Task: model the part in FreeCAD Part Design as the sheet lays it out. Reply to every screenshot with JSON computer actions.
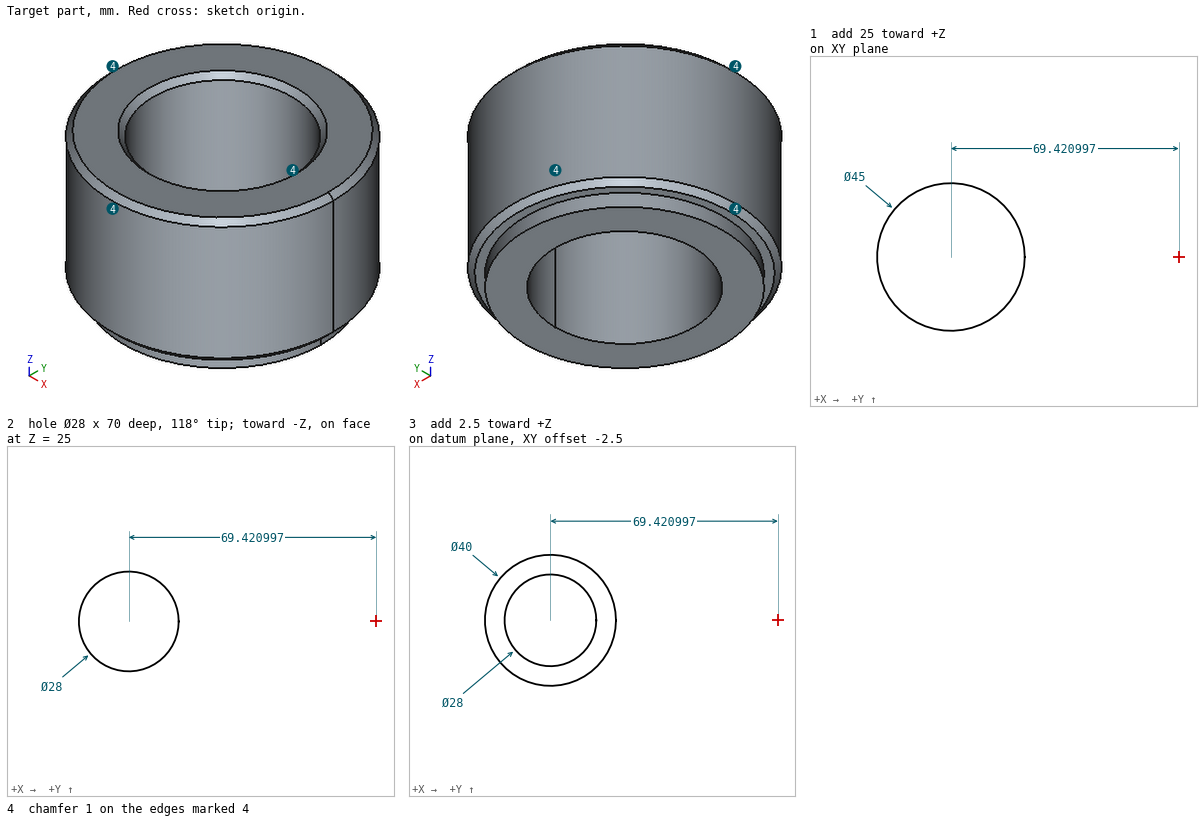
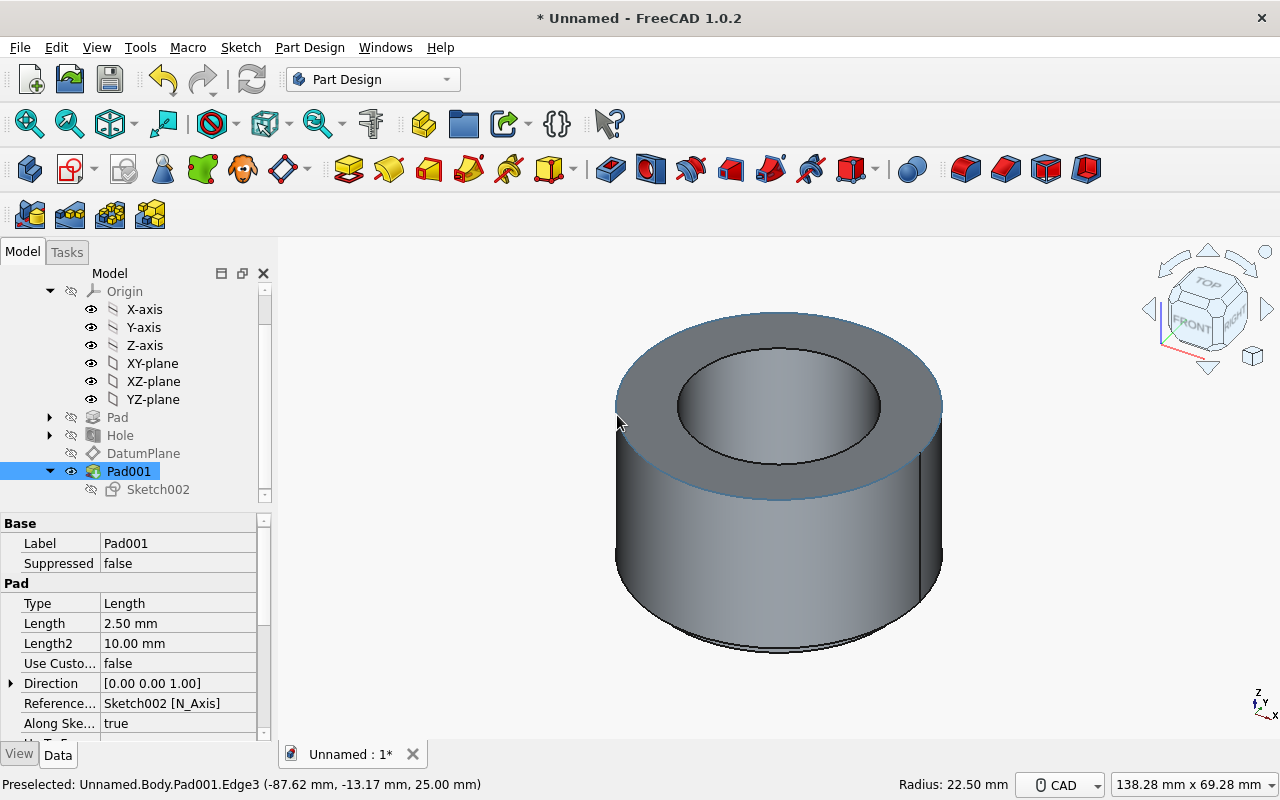
{"action": "left_click", "coordinate": [691, 376], "text": "ctrl"}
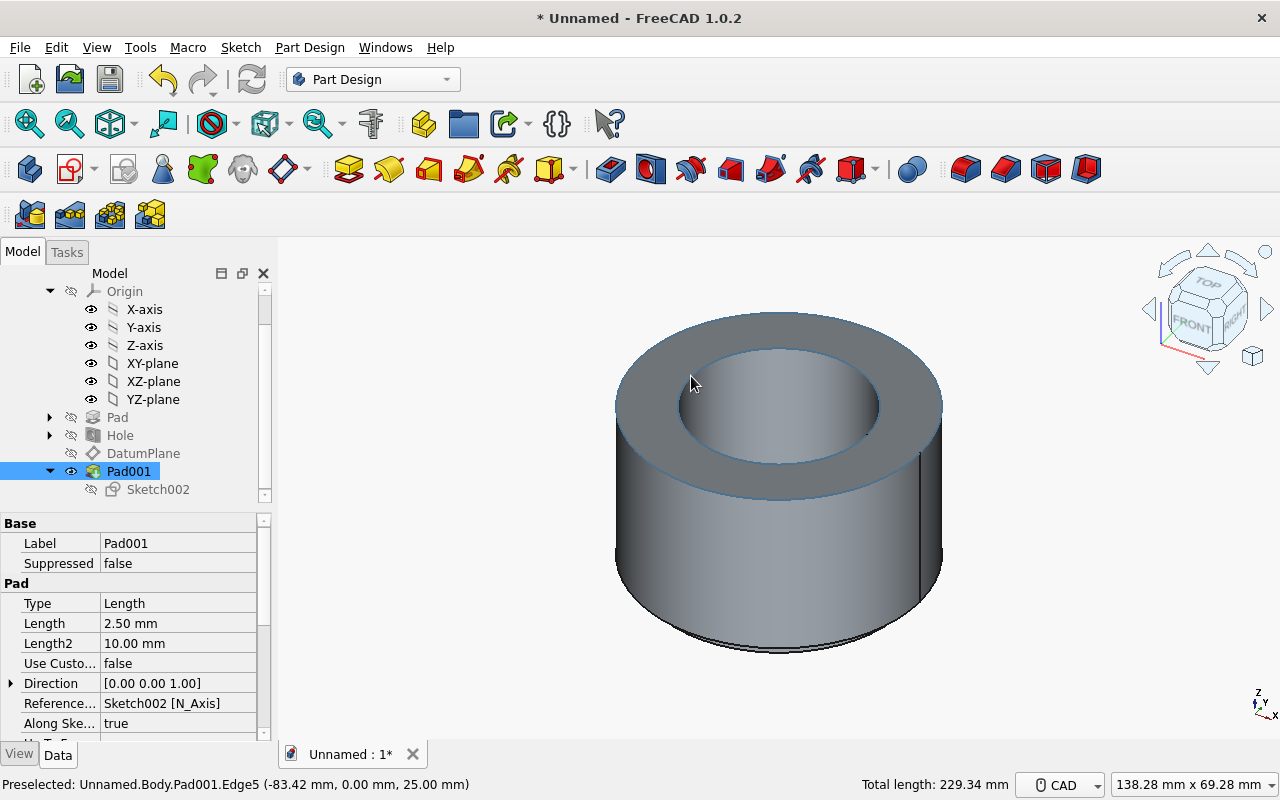
{"action": "key", "text": "0"}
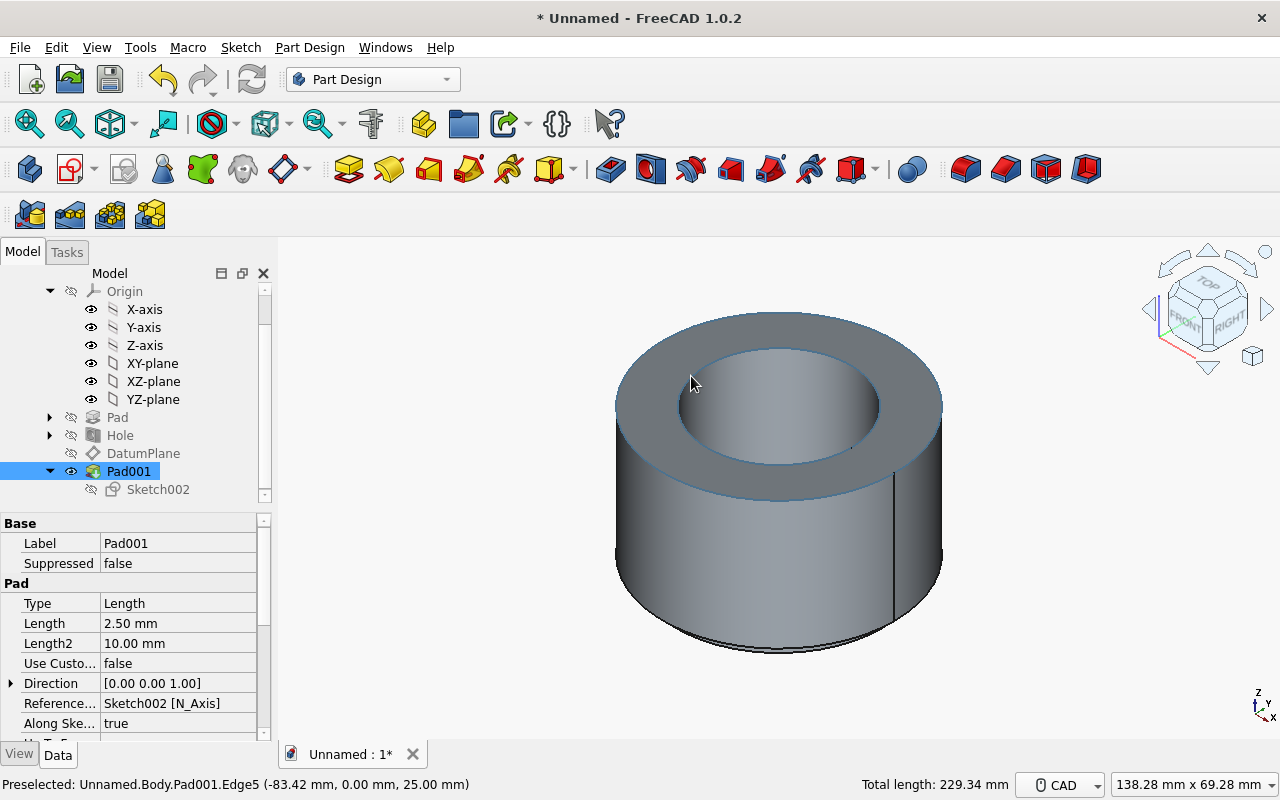
{"action": "key", "text": "2"}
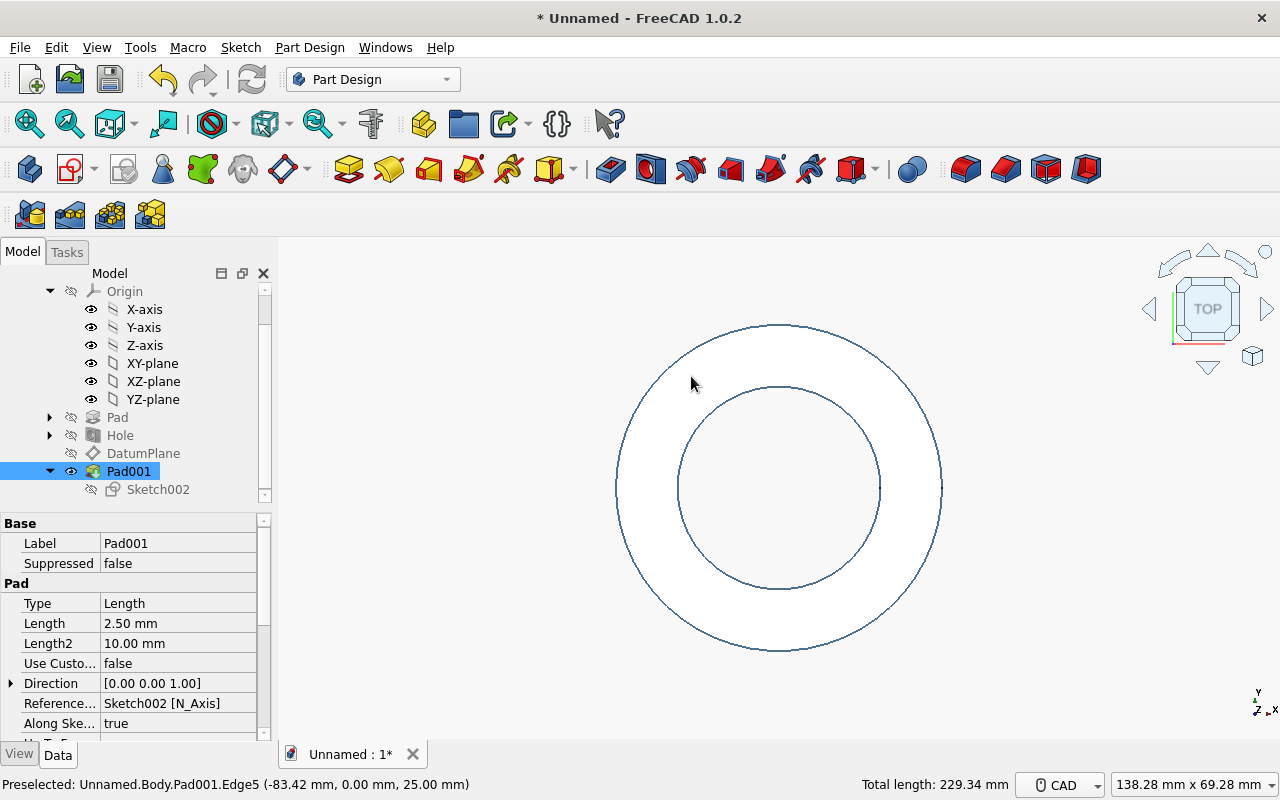
{"action": "key", "text": "1"}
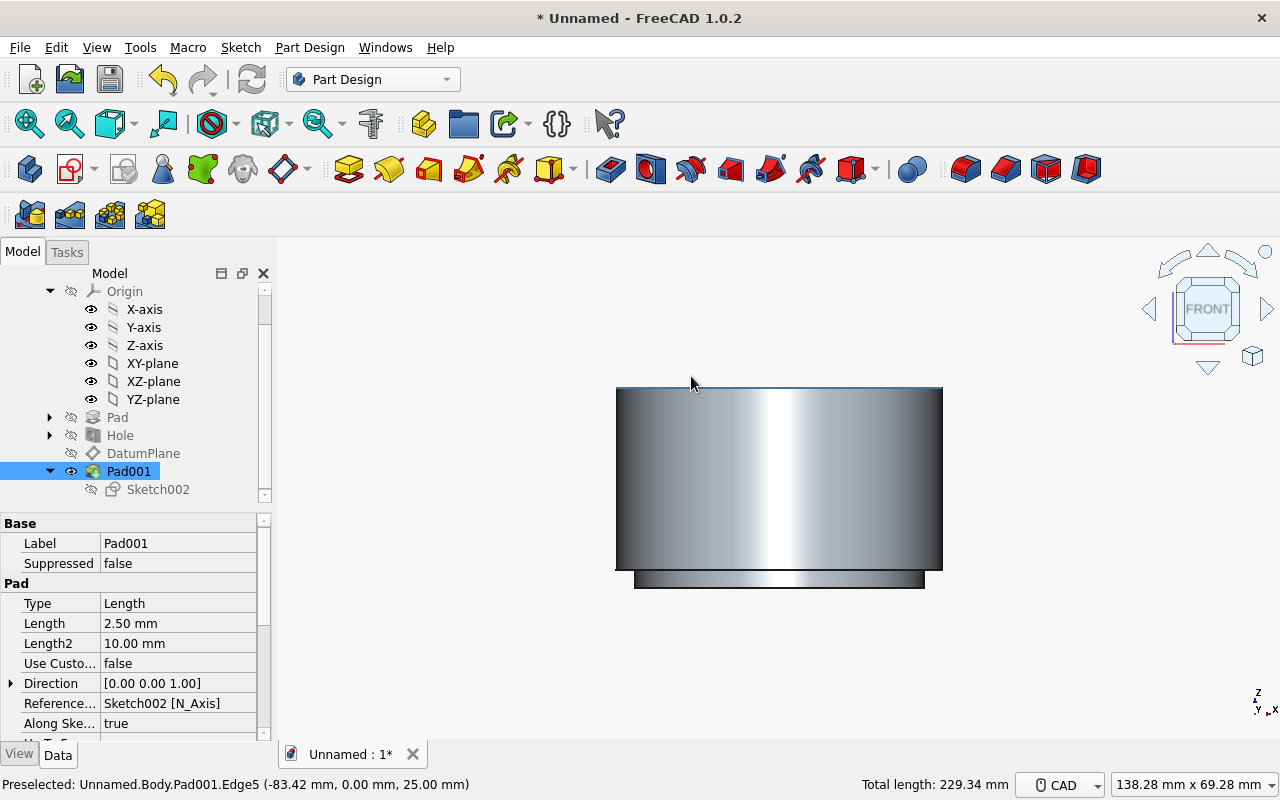
{"action": "left_click", "coordinate": [30, 124]}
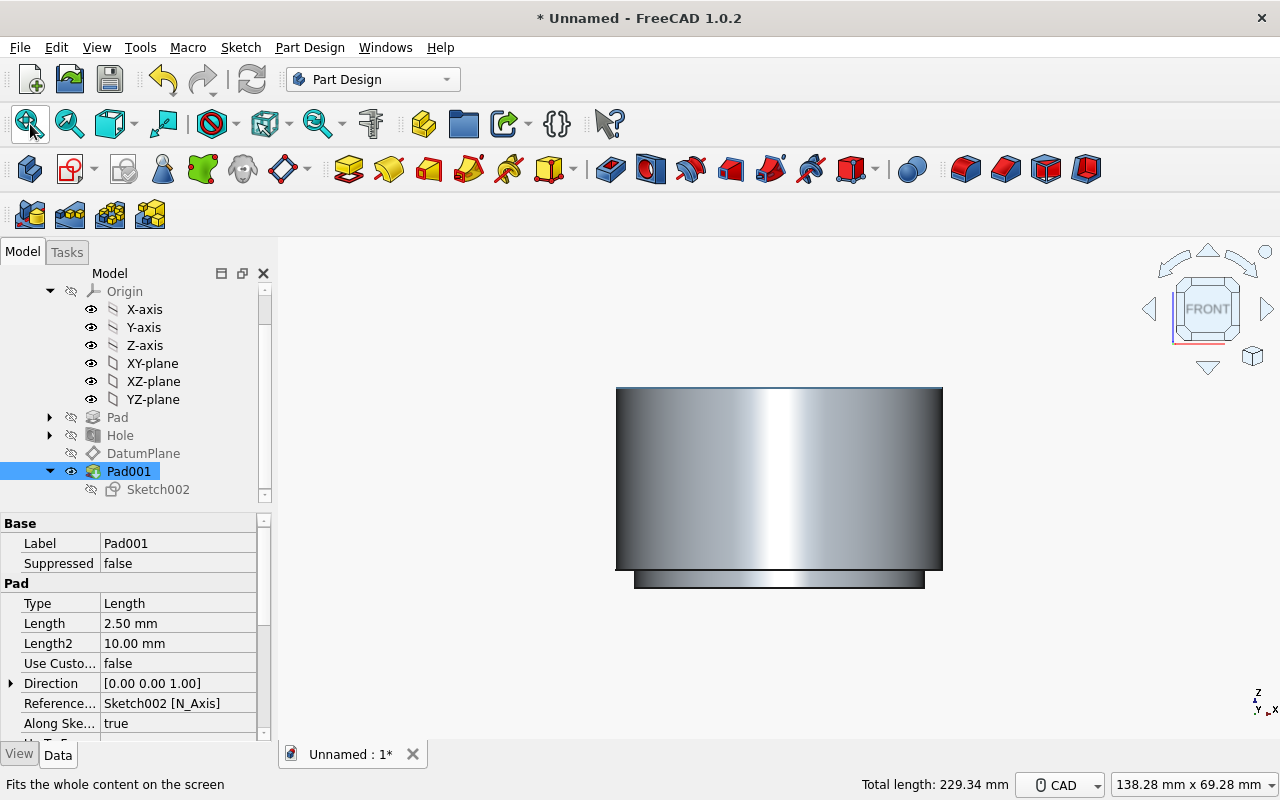
{"action": "left_click", "coordinate": [647, 569], "text": "ctrl"}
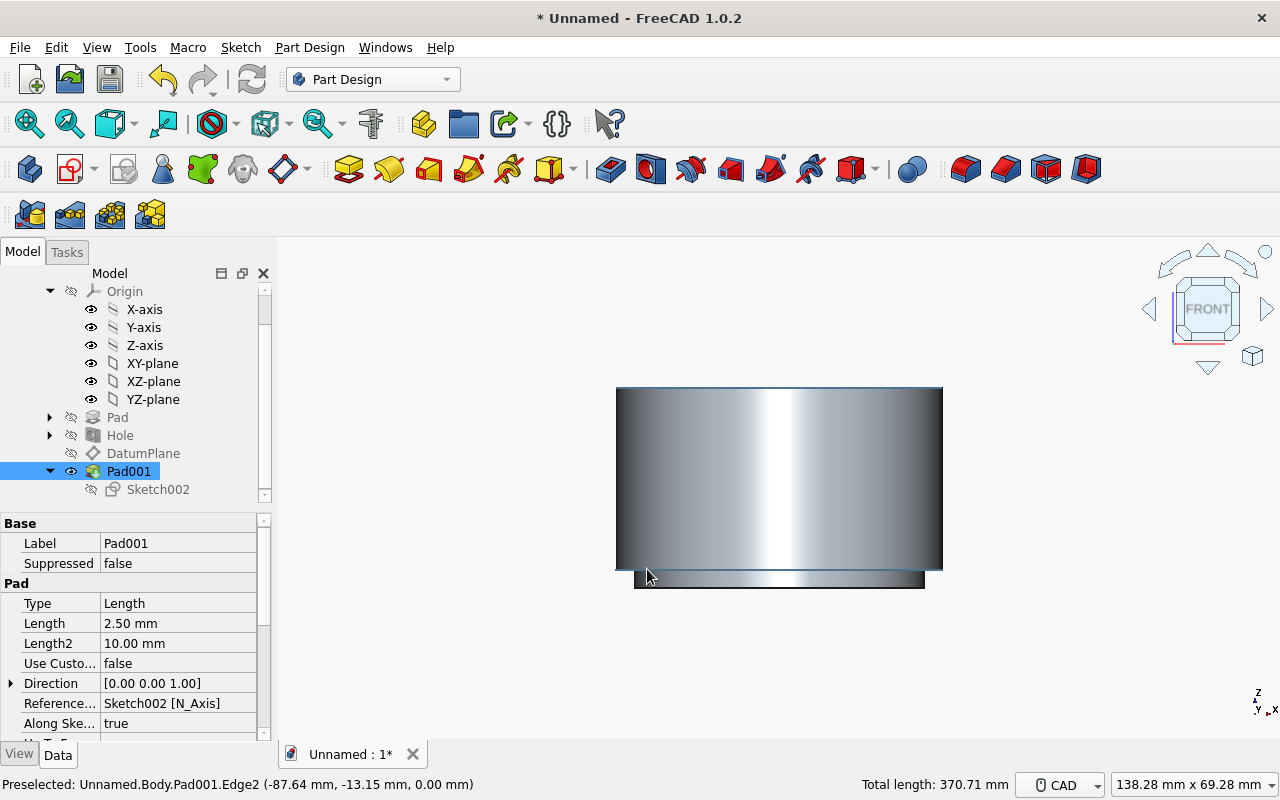
{"action": "left_click", "coordinate": [1006, 170]}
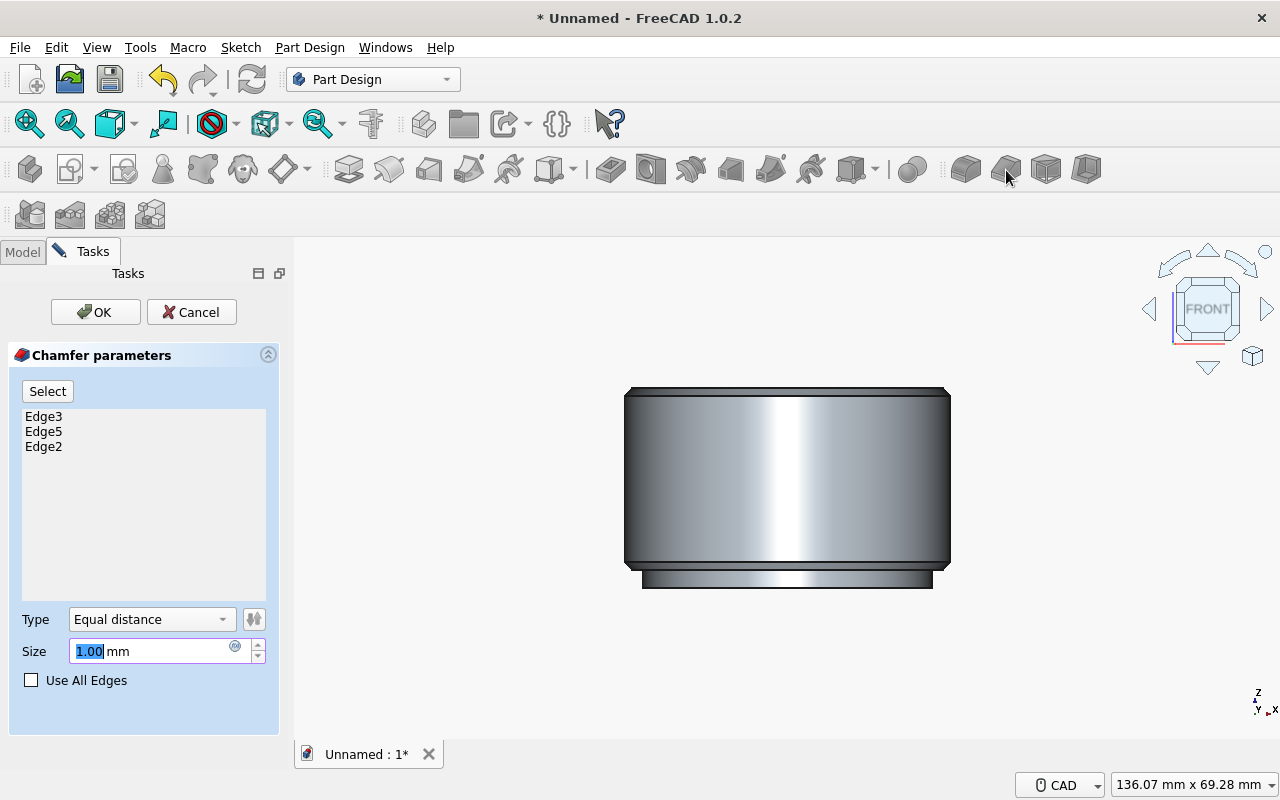
{"action": "type", "text": "1"}
{"action": "key", "text": "Tab"}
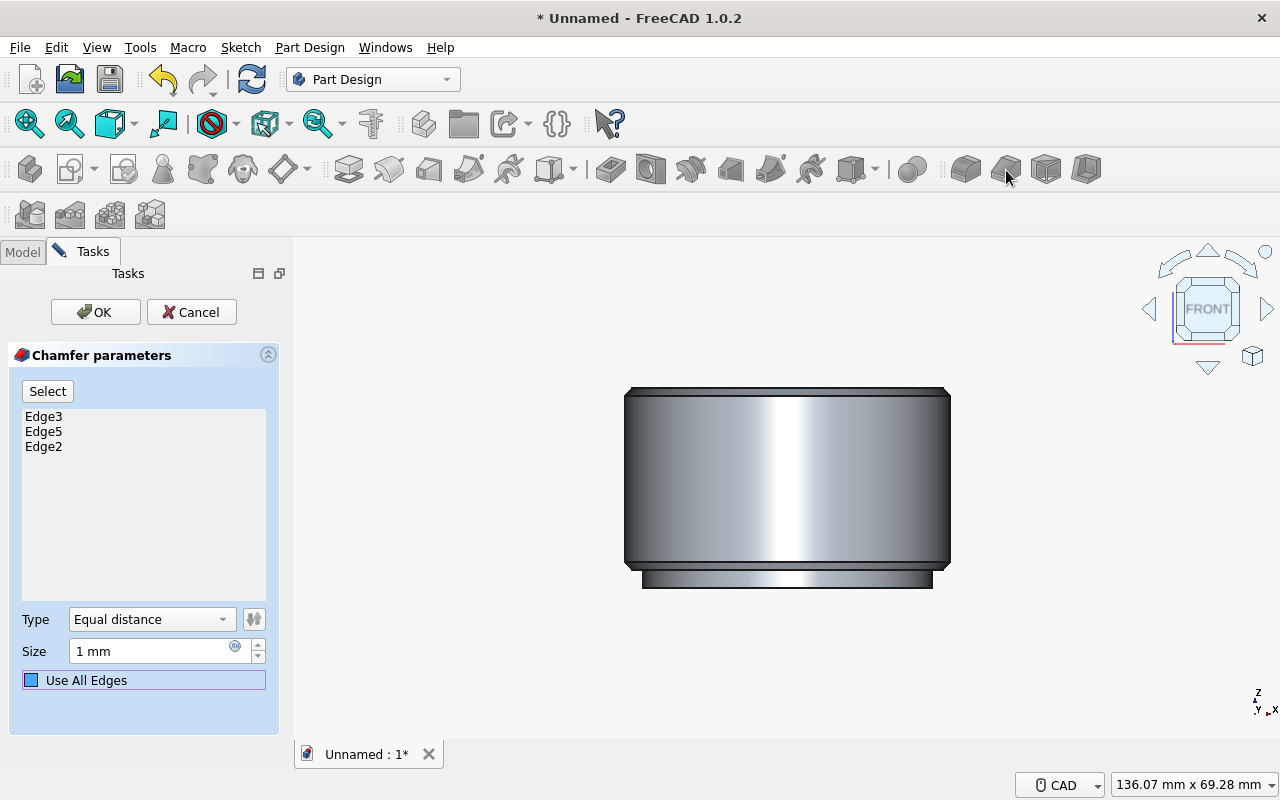
{"action": "left_click", "coordinate": [96, 312]}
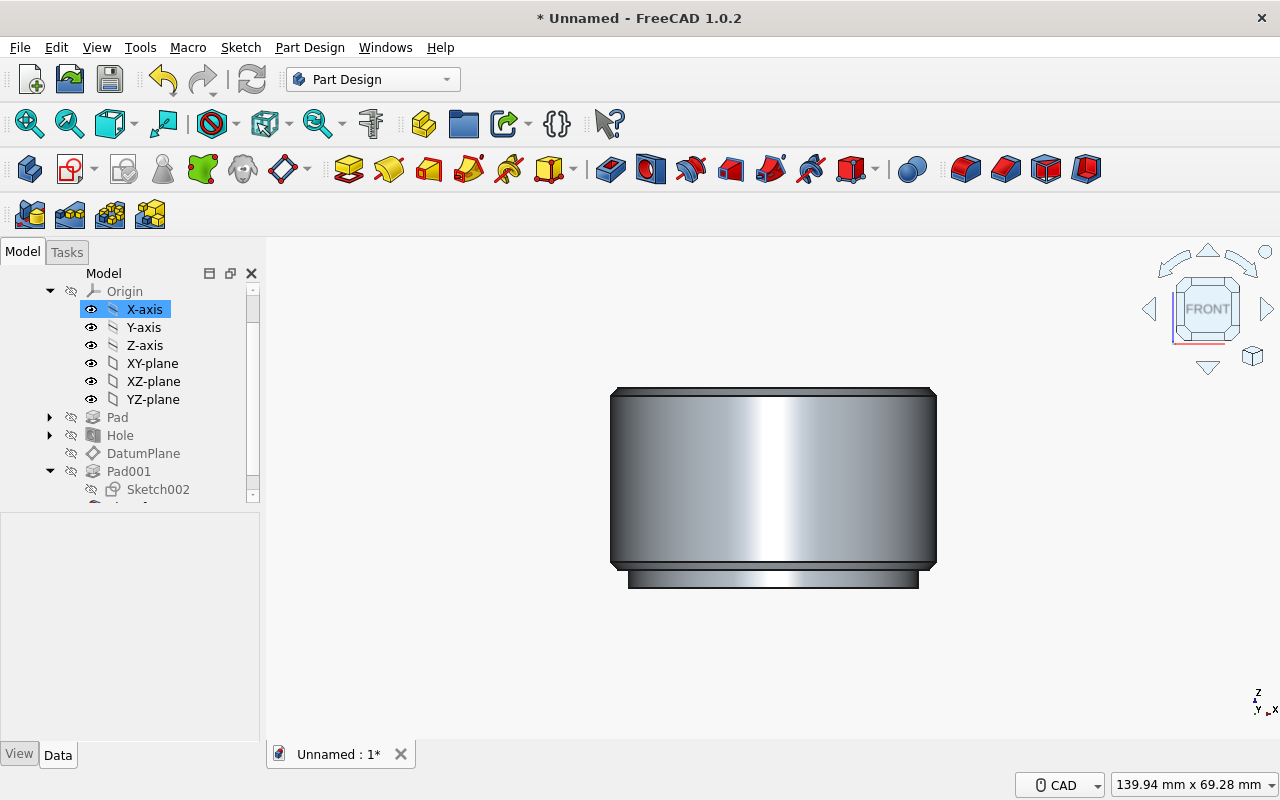
{"action": "key", "text": "0"}